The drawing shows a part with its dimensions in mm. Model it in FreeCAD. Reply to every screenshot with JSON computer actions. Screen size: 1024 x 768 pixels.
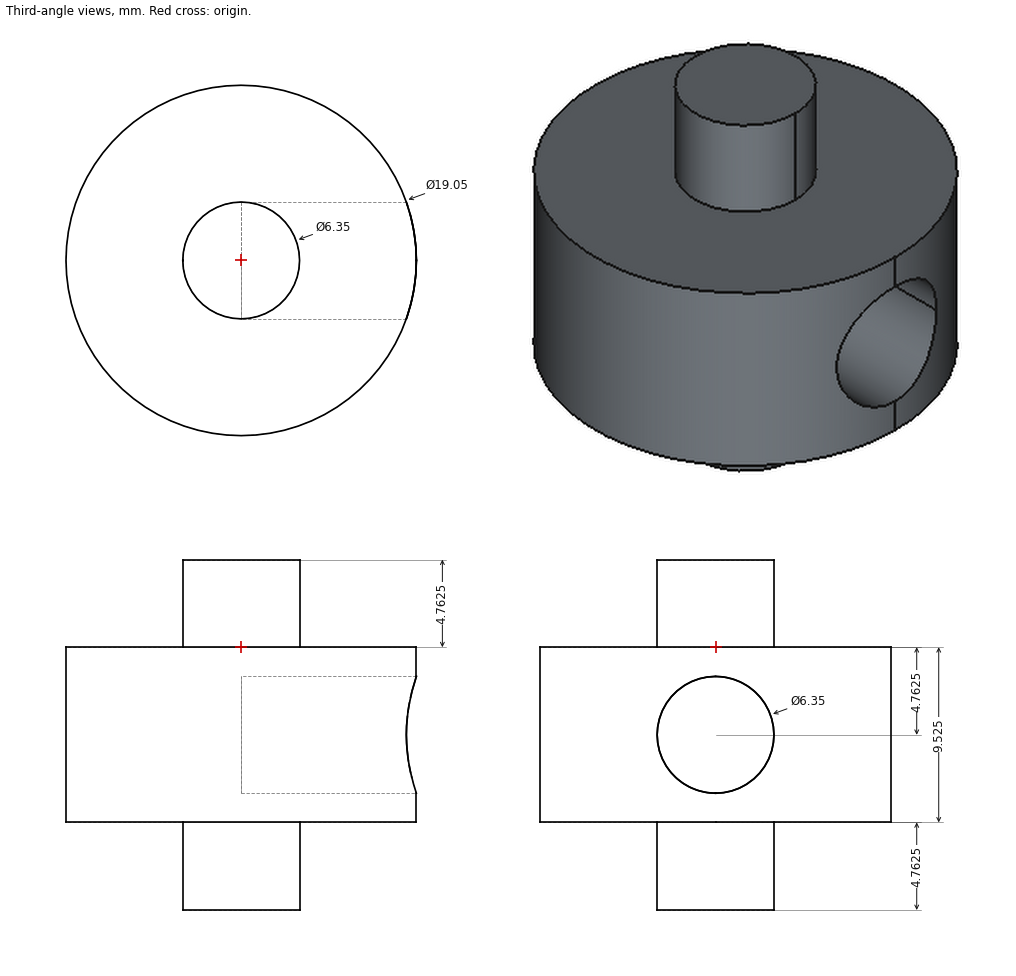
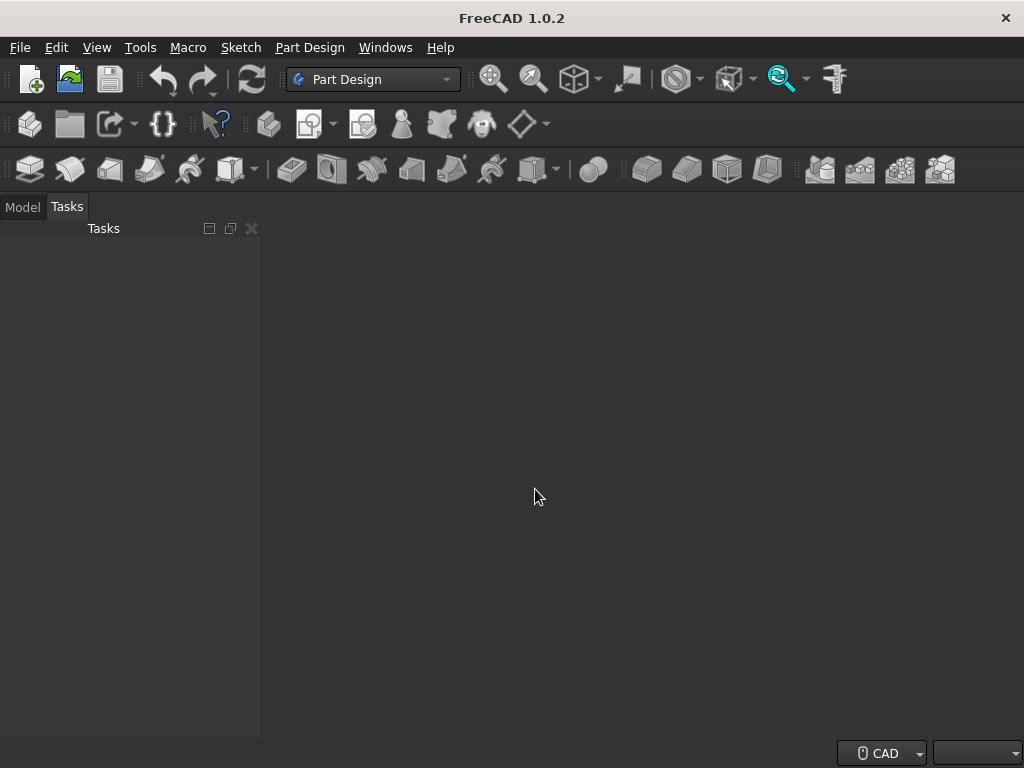
{"action": "left_click", "coordinate": [30, 80]}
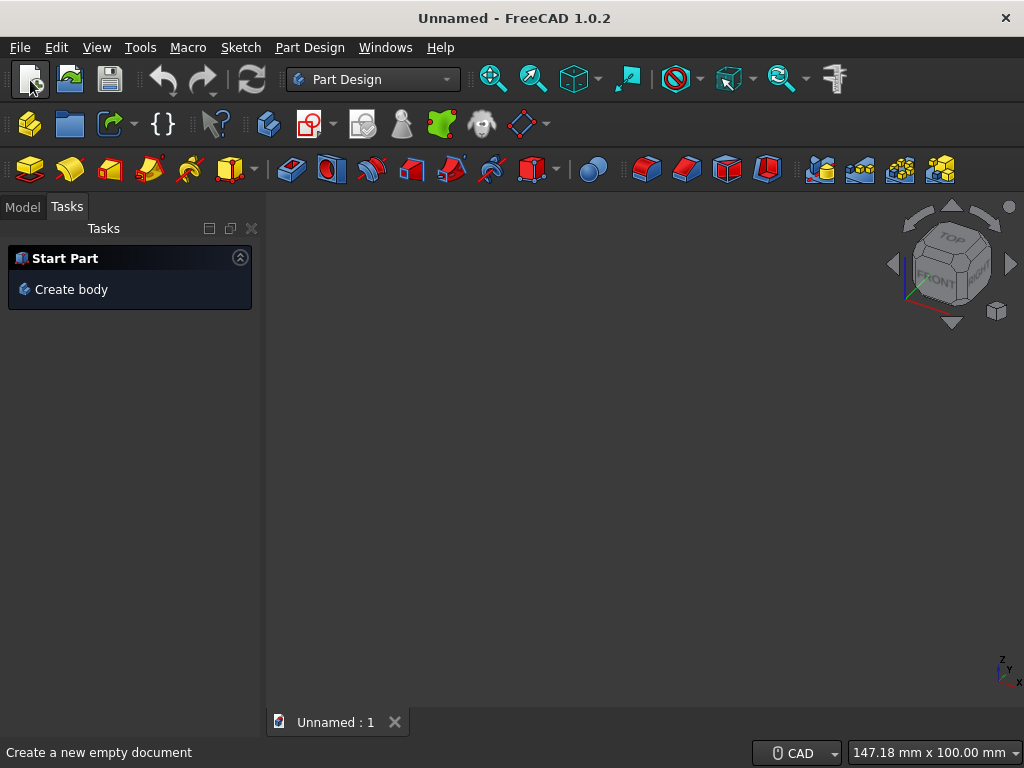
{"action": "left_click", "coordinate": [310, 124]}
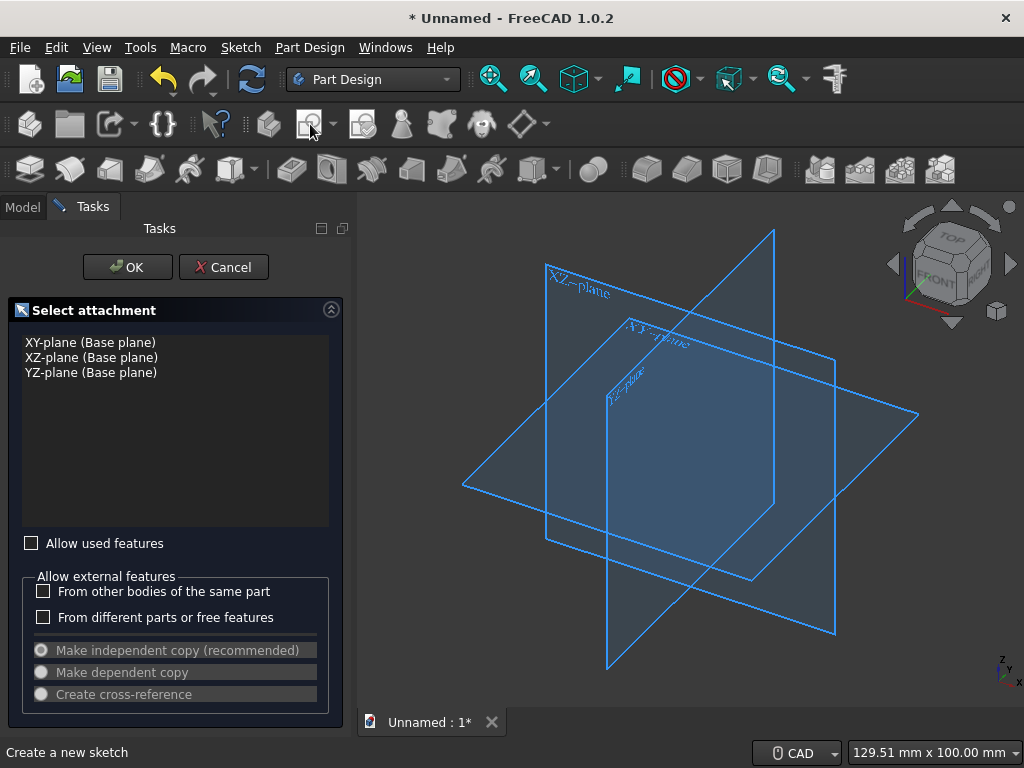
{"action": "left_click", "coordinate": [82, 342]}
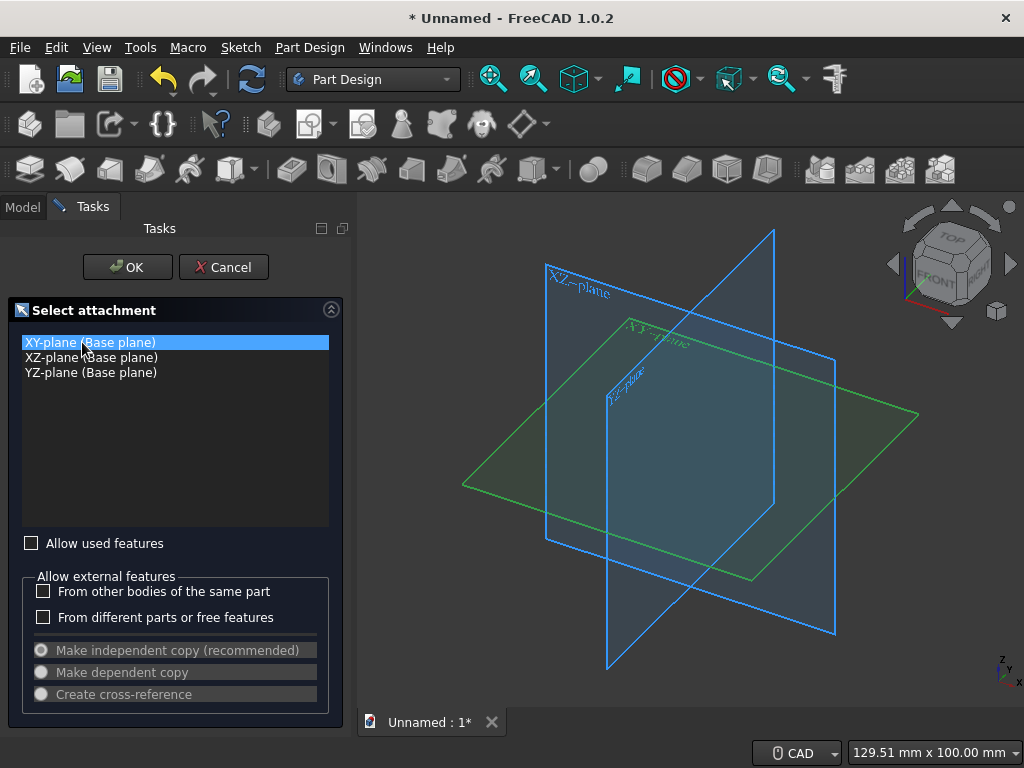
{"action": "left_click", "coordinate": [128, 267]}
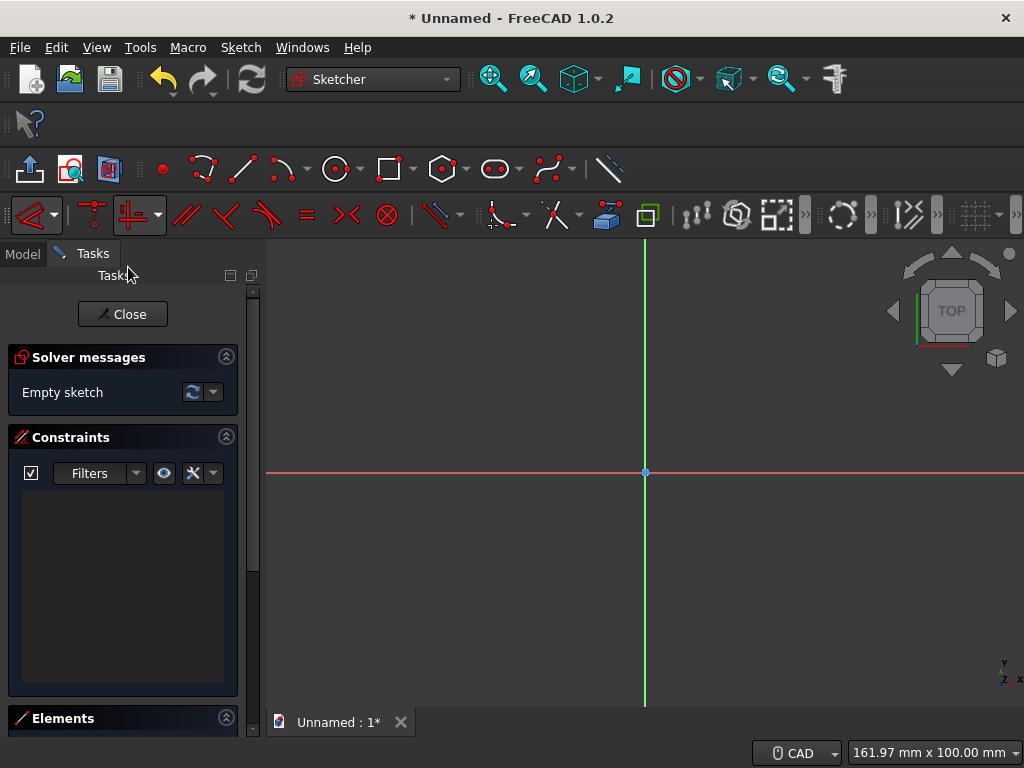
{"action": "scroll", "coordinate": [675, 473], "scroll_direction": "up", "scroll_amount": 6}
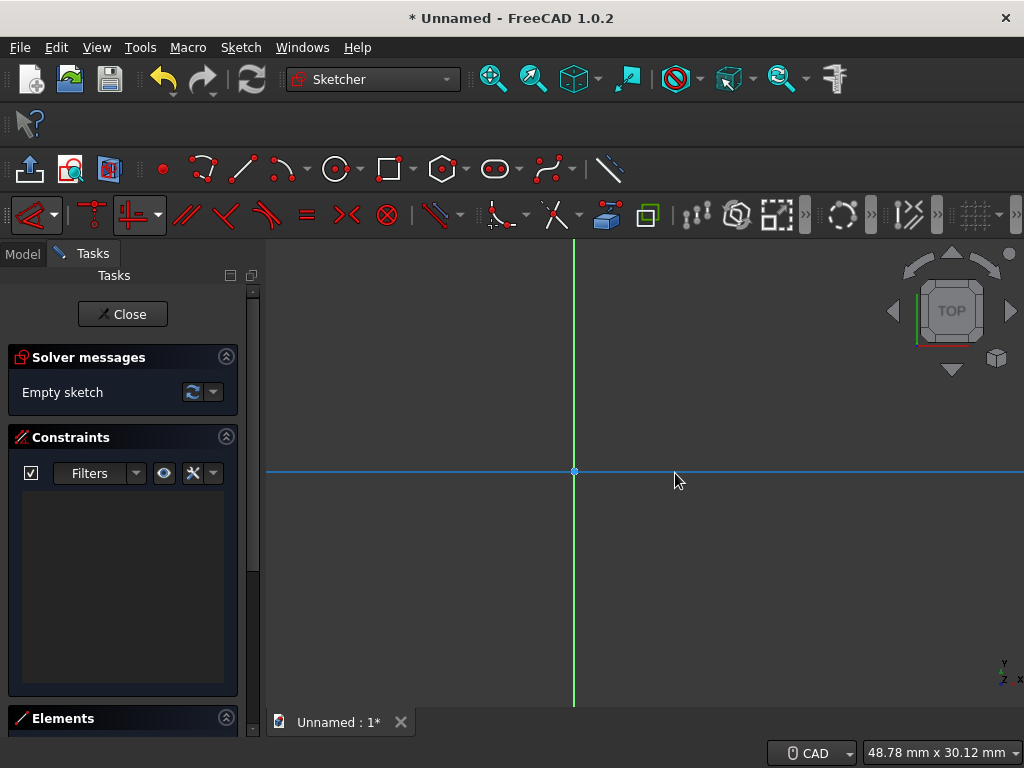
{"action": "key", "text": "g c"}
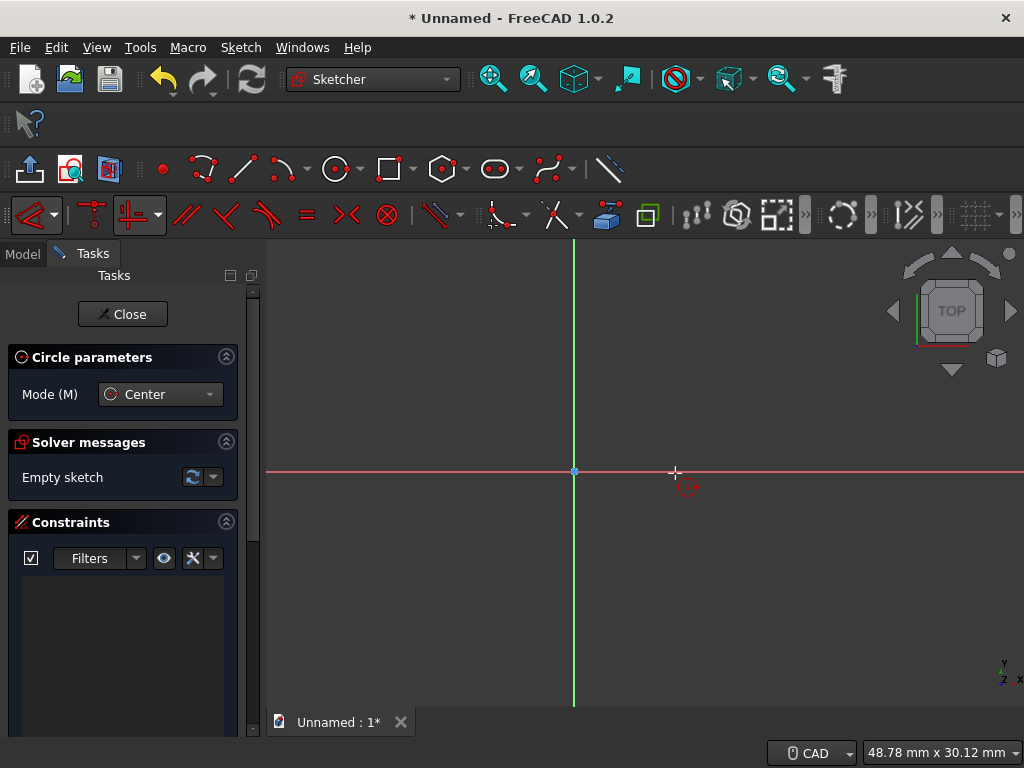
{"action": "left_click", "coordinate": [574, 472]}
{"action": "left_click", "coordinate": [679, 367]}
{"action": "key", "text": "Escape"}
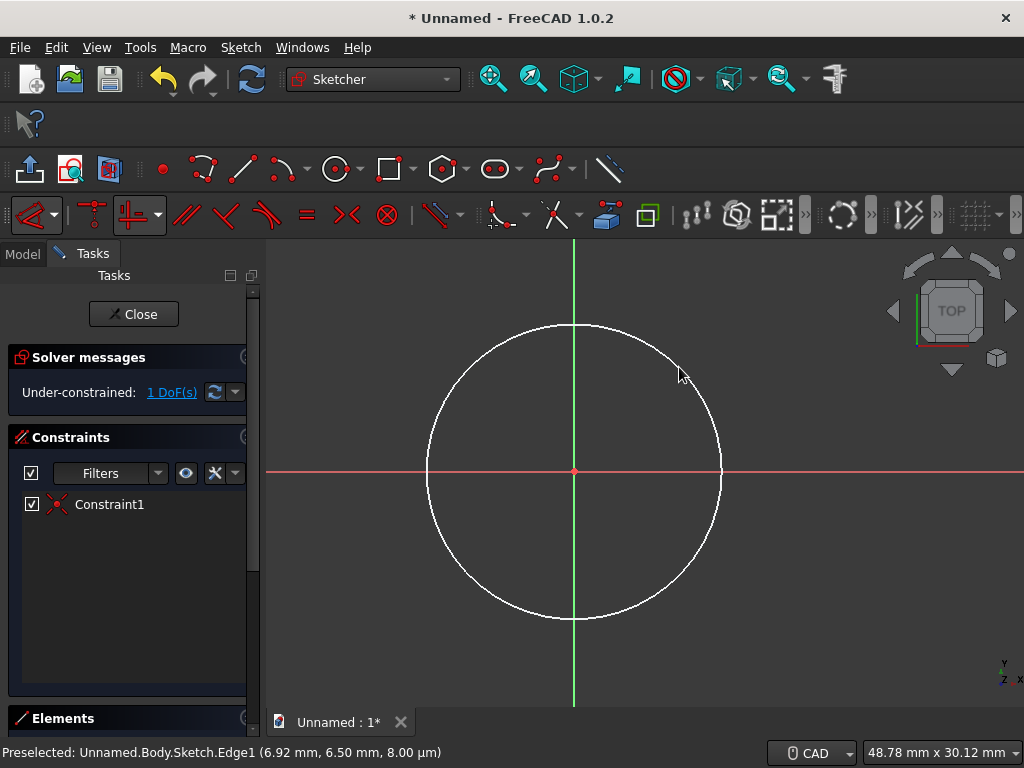
{"action": "left_click", "coordinate": [678, 367]}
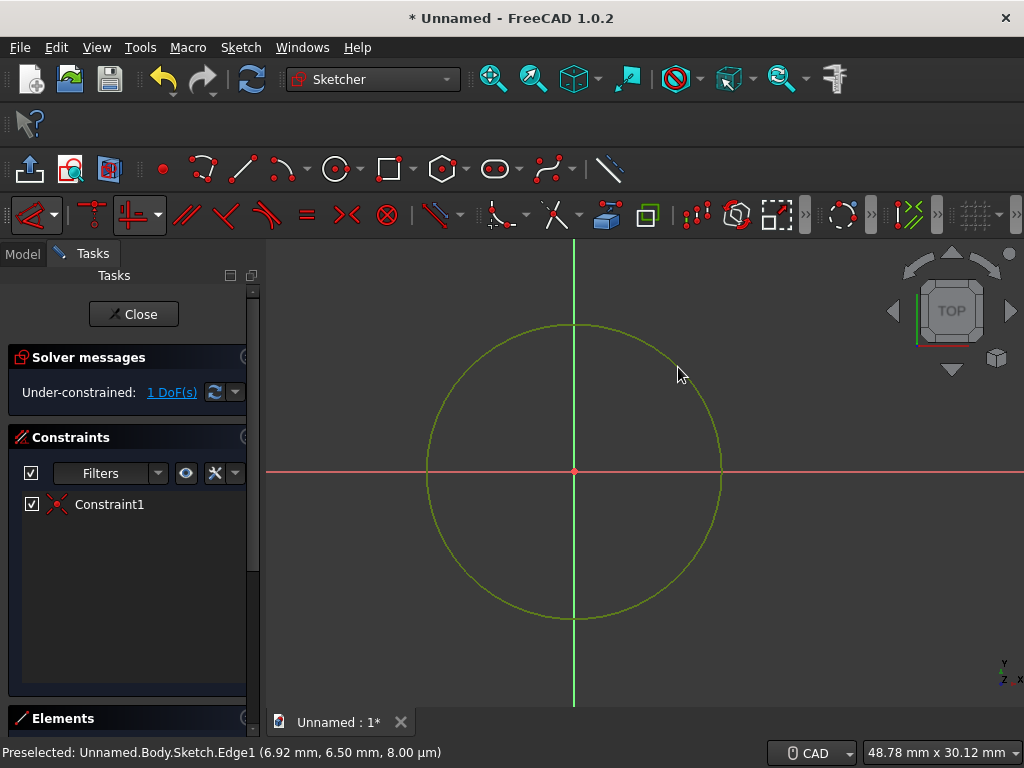
{"action": "left_click", "coordinate": [56, 216]}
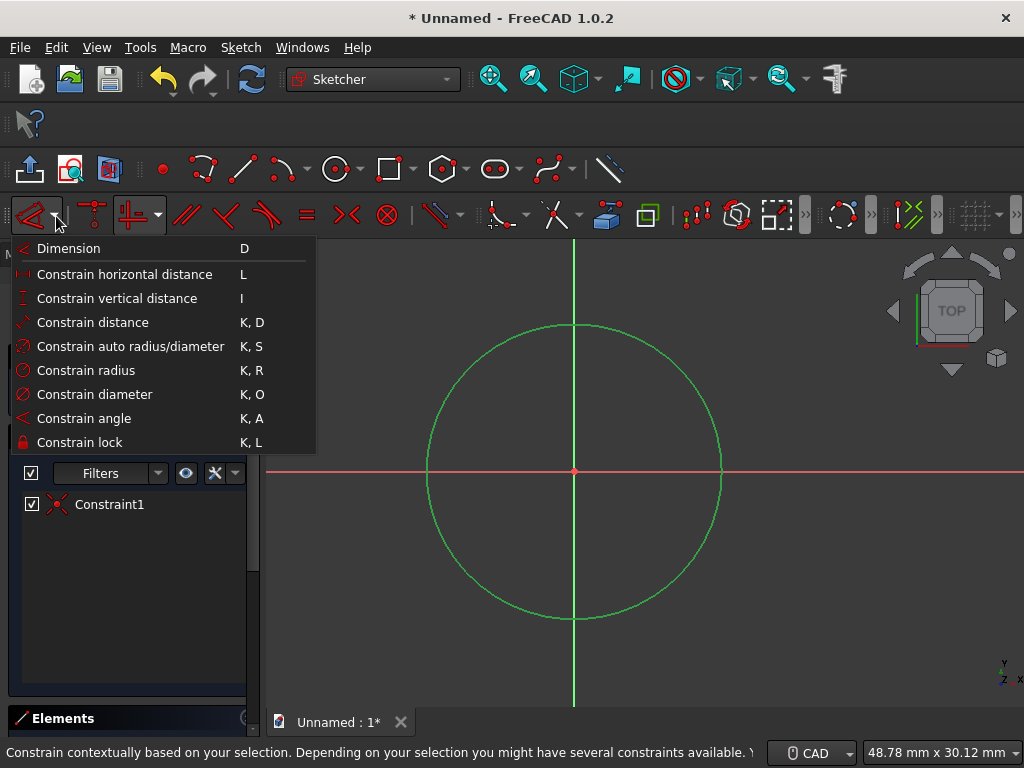
{"action": "left_click", "coordinate": [164, 394]}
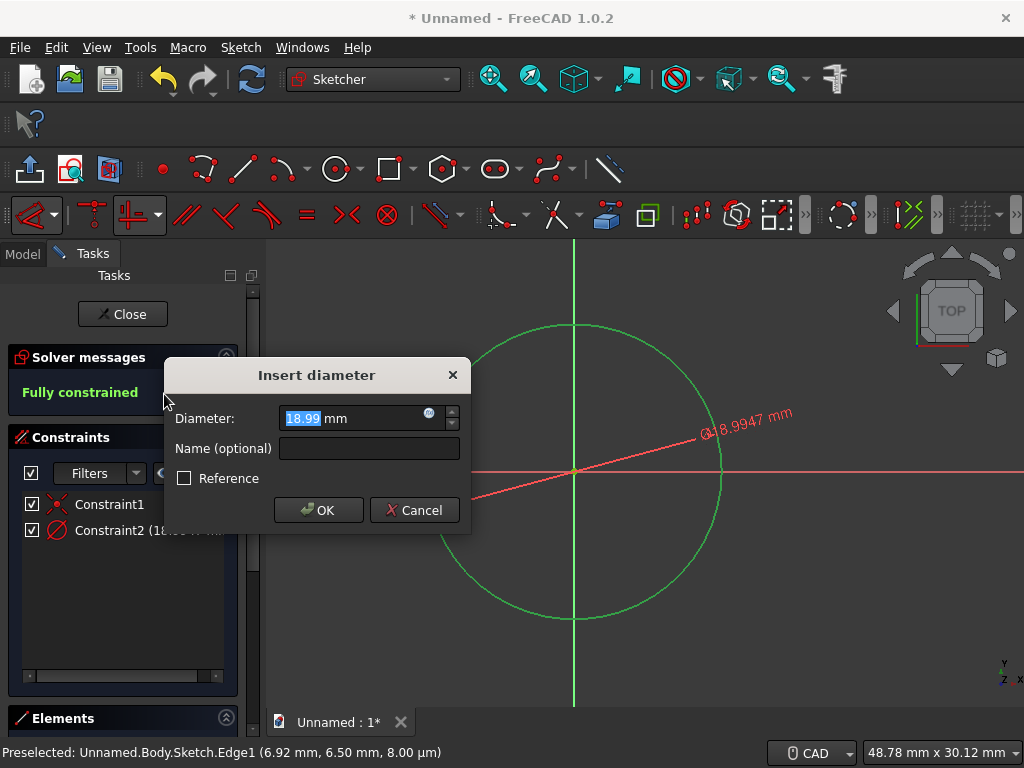
{"action": "type", "text": "19.05"}
{"action": "key", "text": "Return"}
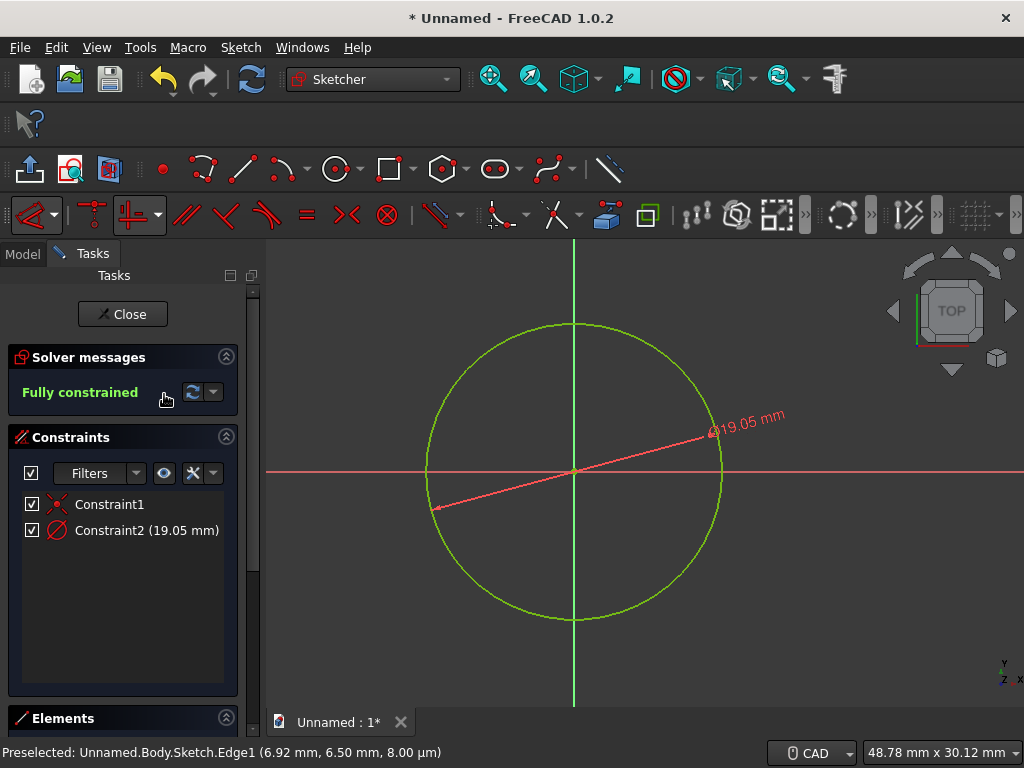
{"action": "left_click", "coordinate": [123, 314]}